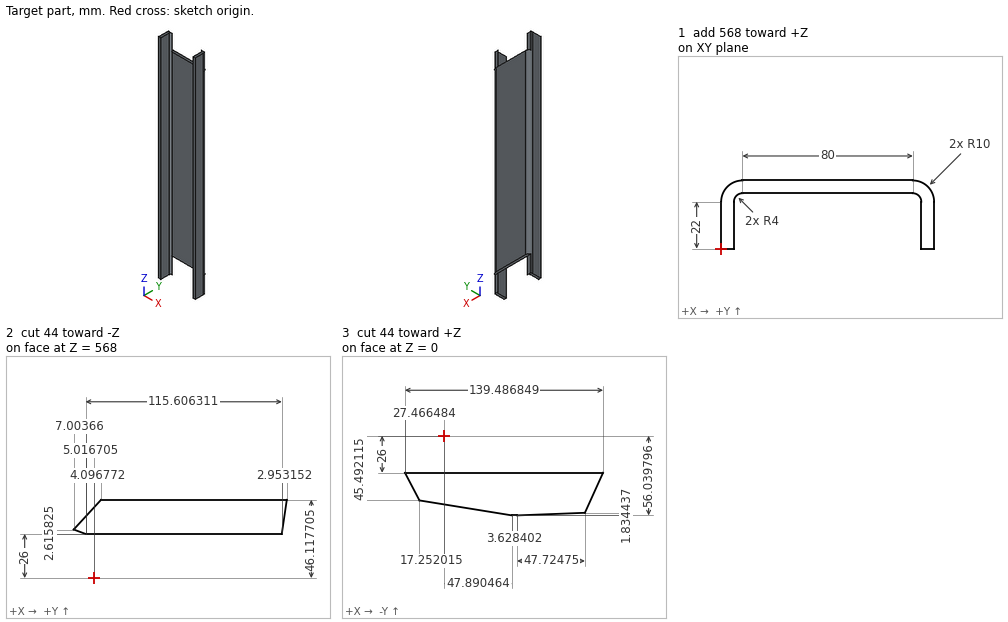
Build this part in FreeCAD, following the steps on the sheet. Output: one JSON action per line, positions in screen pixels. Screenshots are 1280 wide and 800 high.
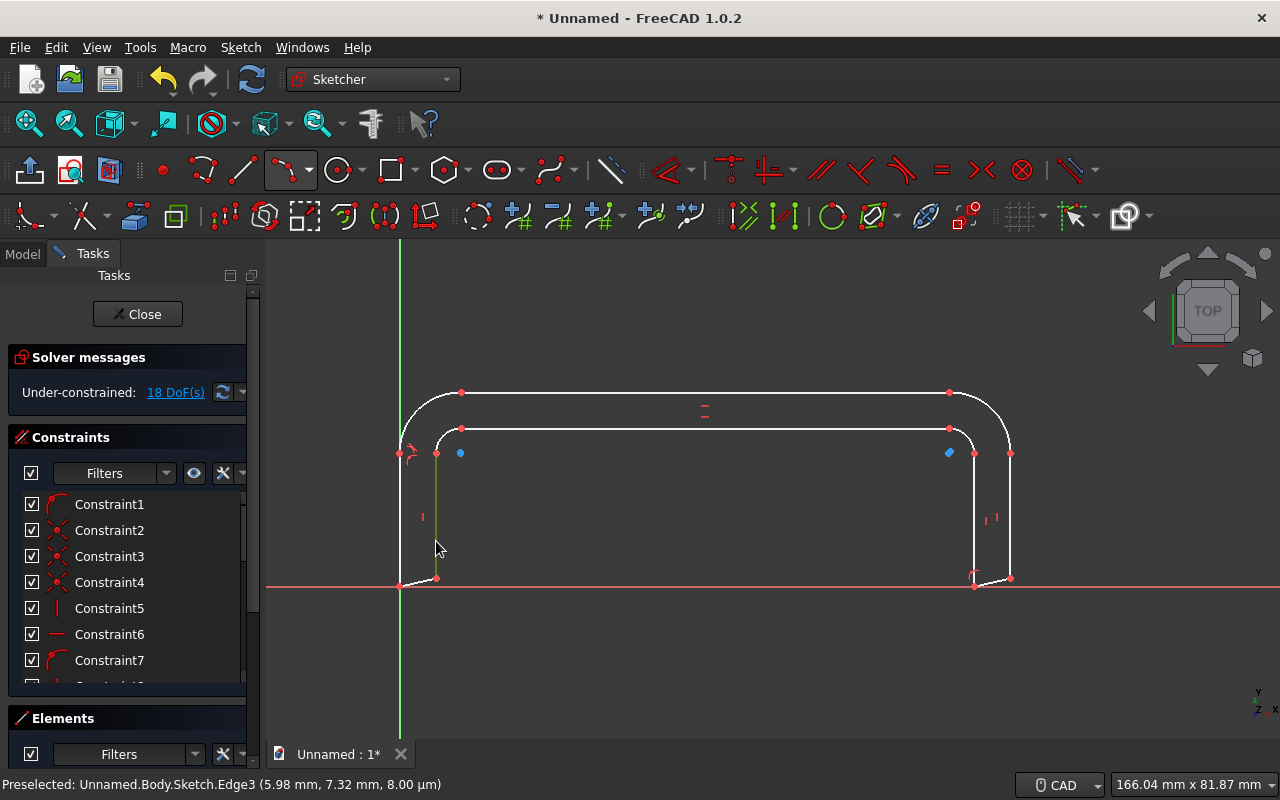
{"action": "left_click", "coordinate": [450, 431]}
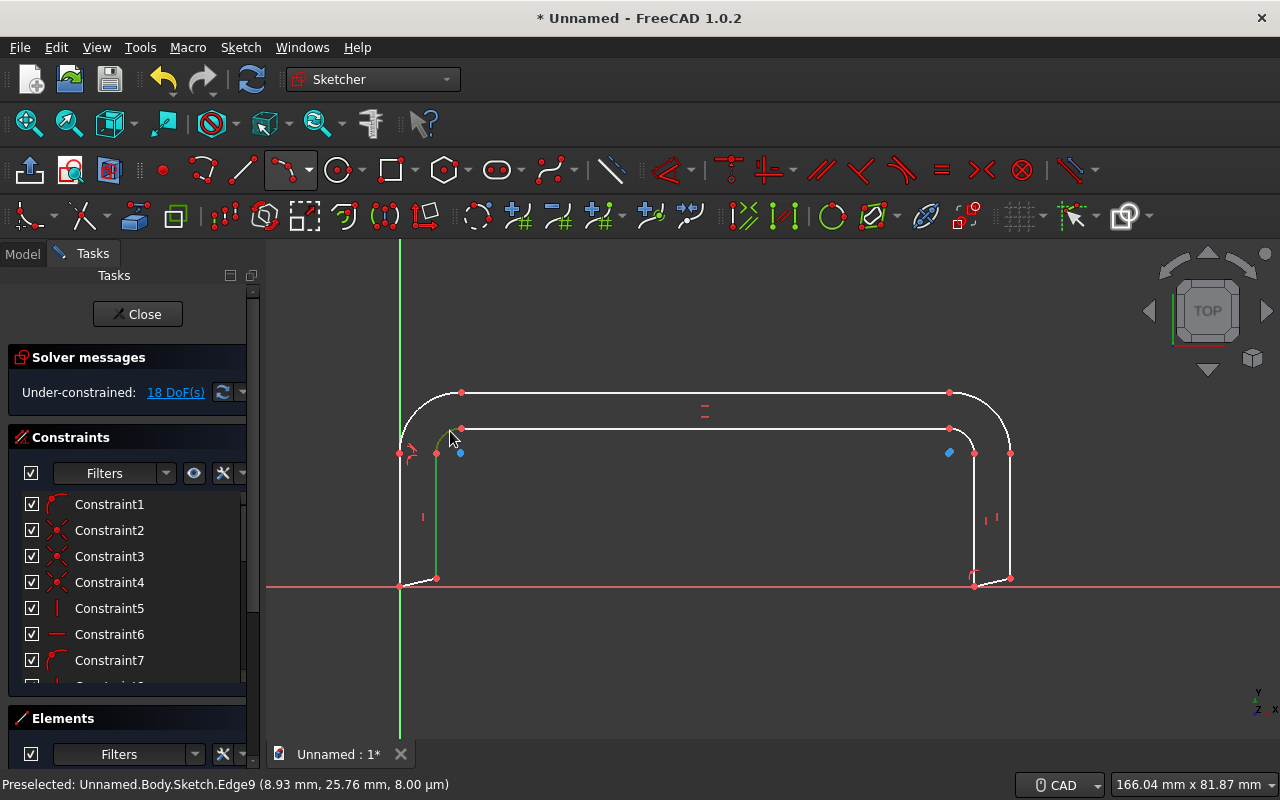
{"action": "left_click", "coordinate": [902, 170]}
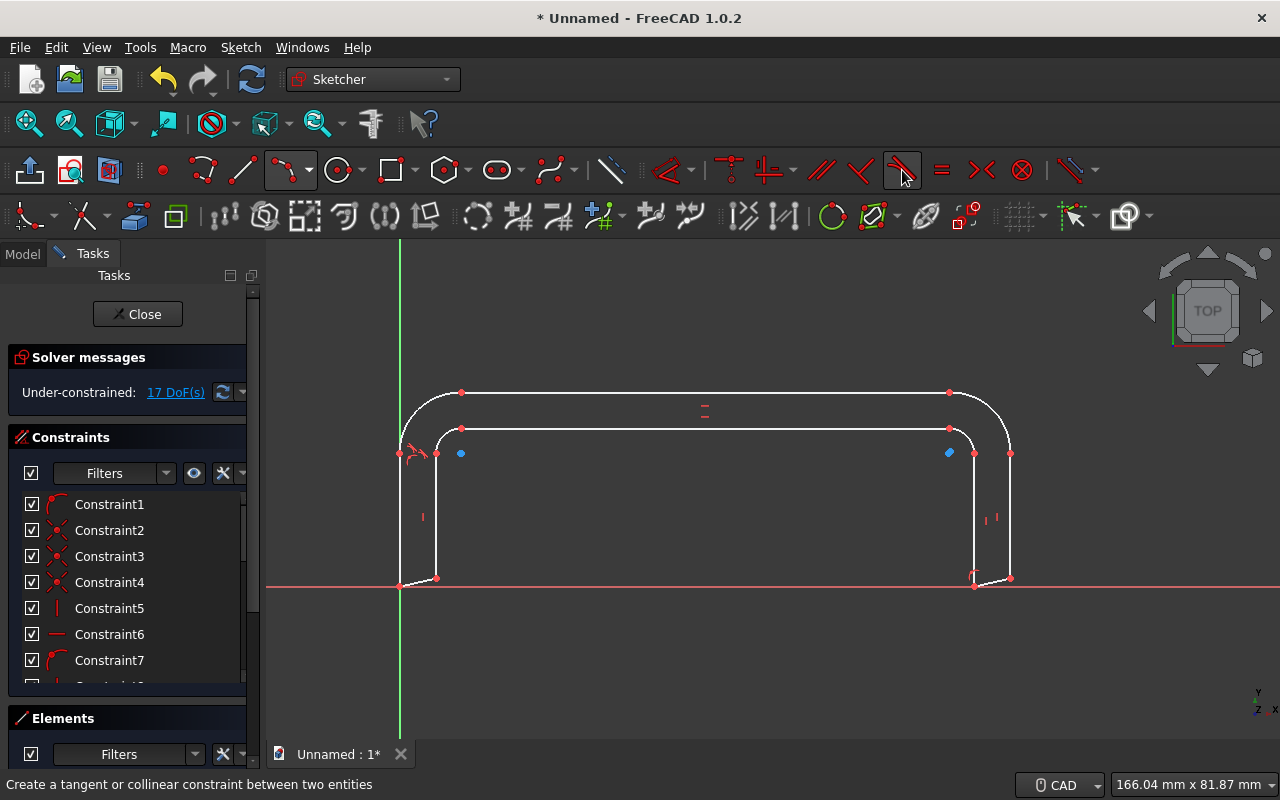
{"action": "left_click", "coordinate": [608, 429]}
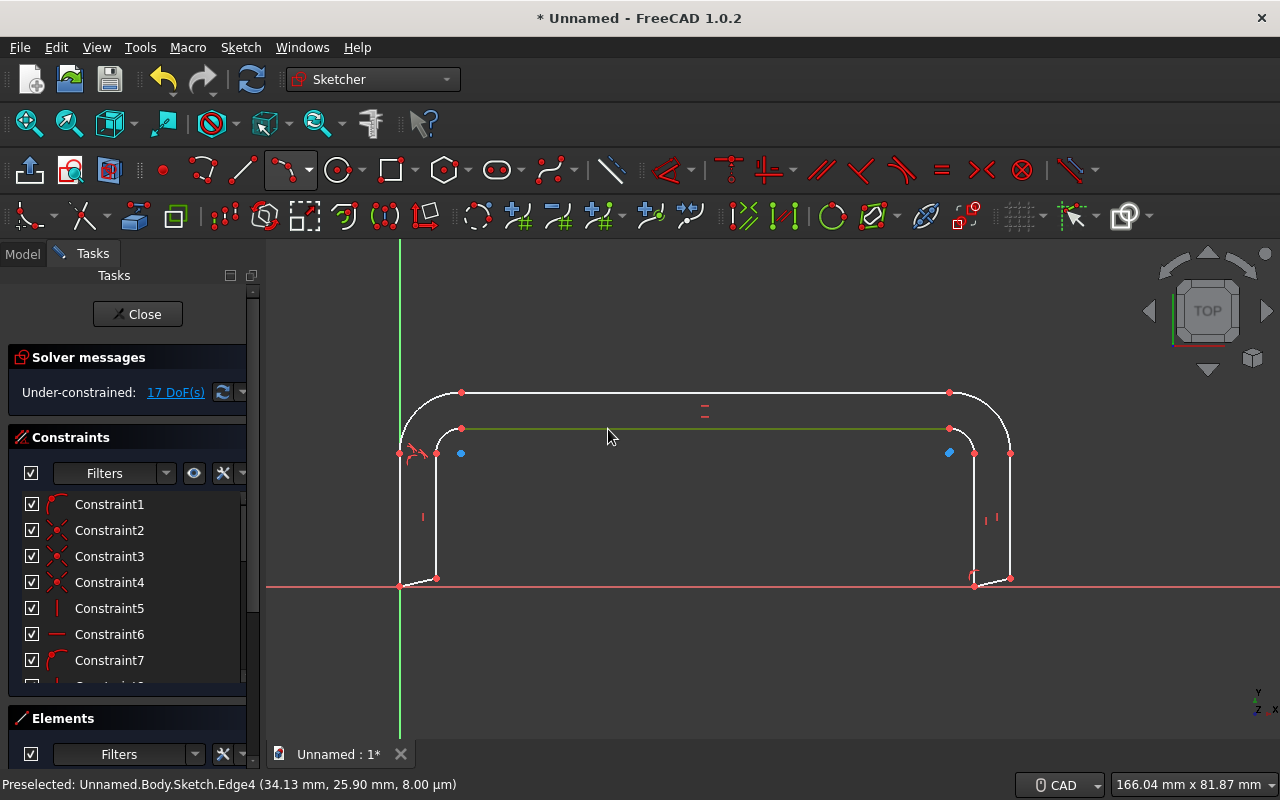
{"action": "left_click", "coordinate": [450, 431]}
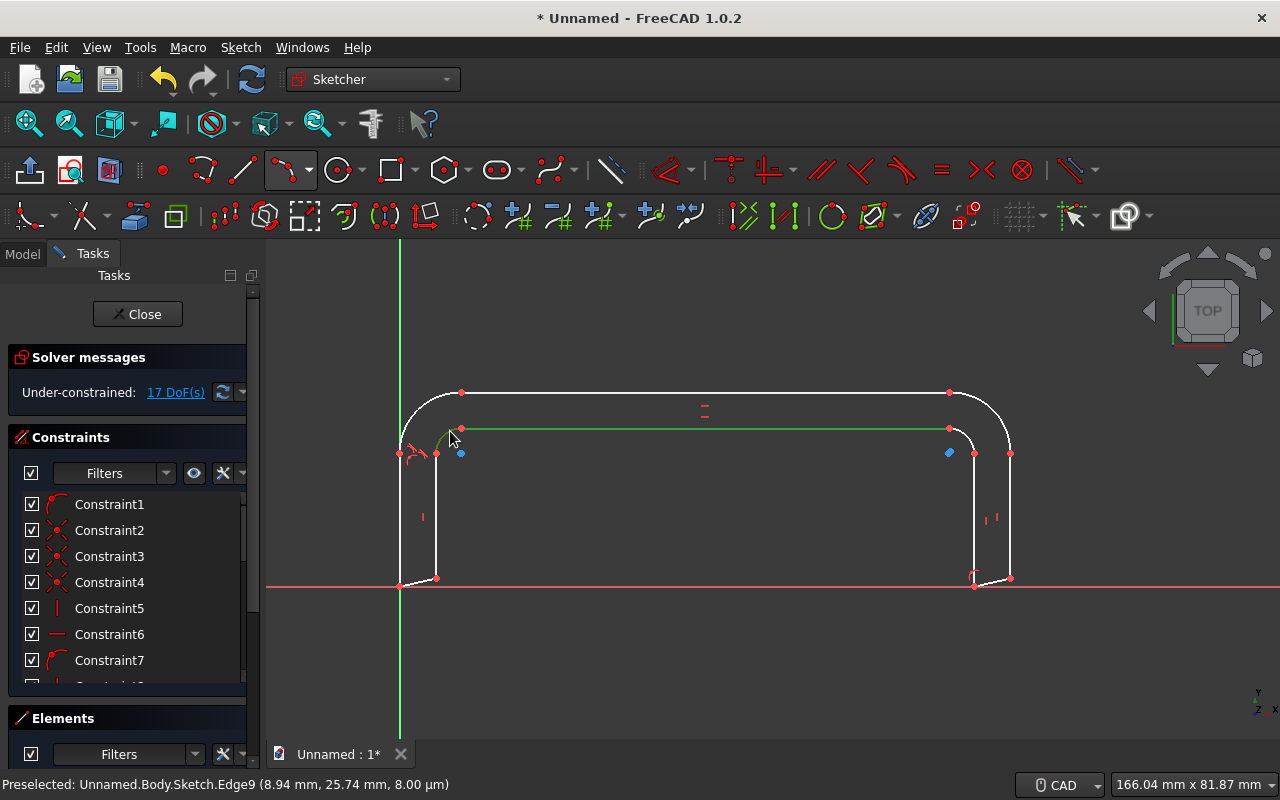
{"action": "left_click", "coordinate": [902, 170]}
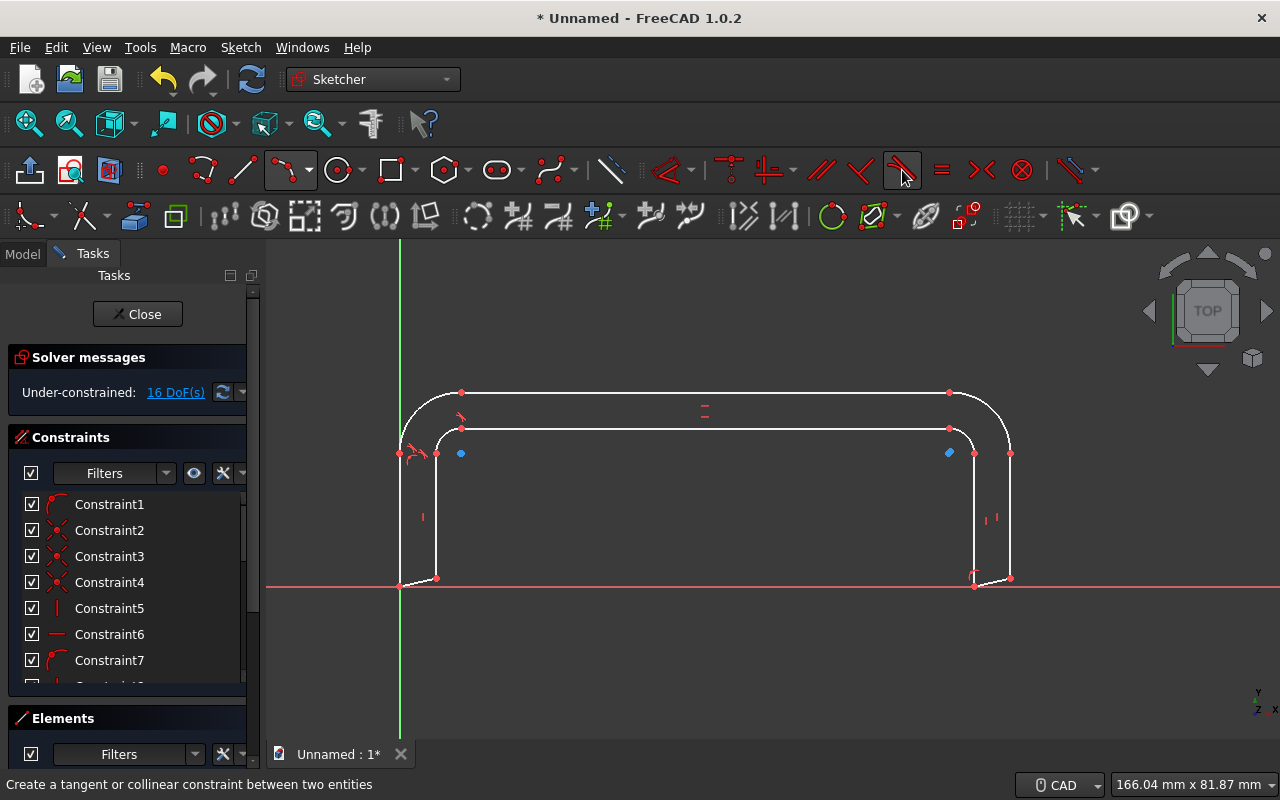
{"action": "left_click", "coordinate": [608, 429]}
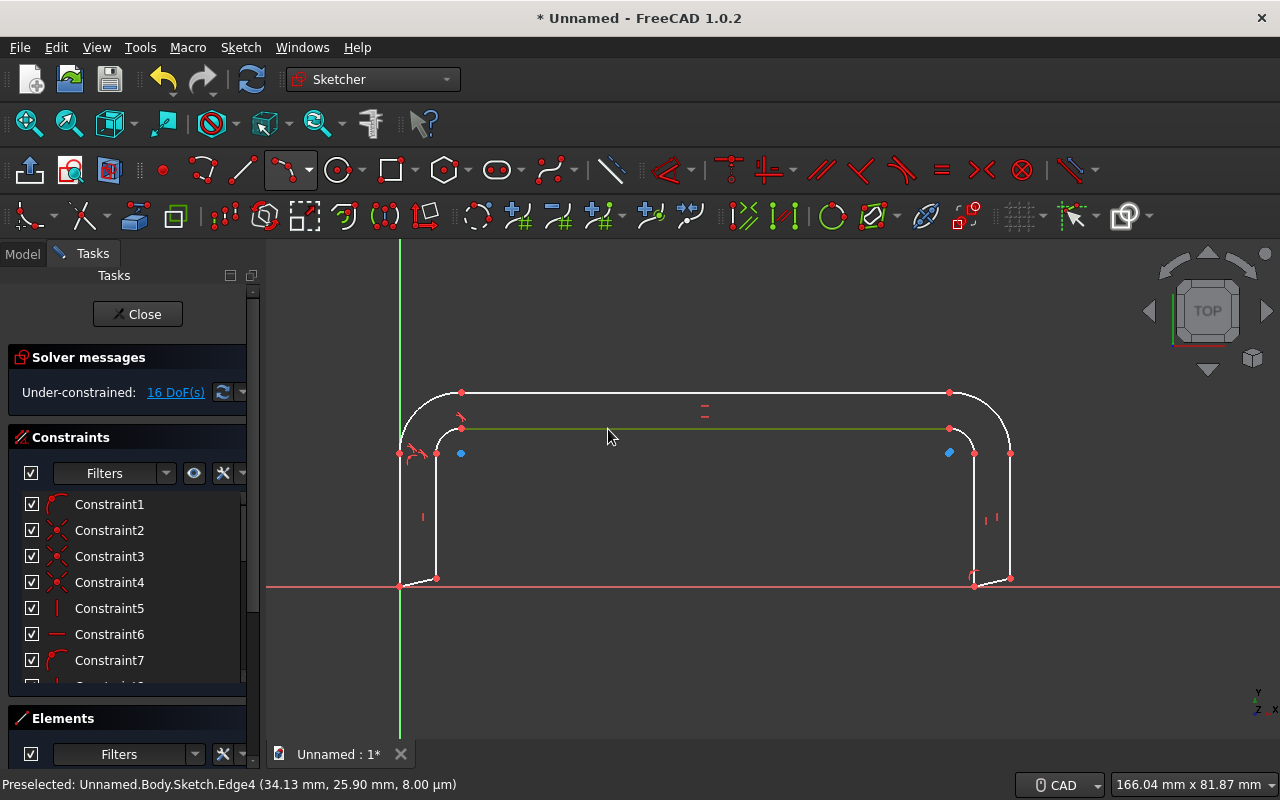
{"action": "left_click", "coordinate": [971, 442]}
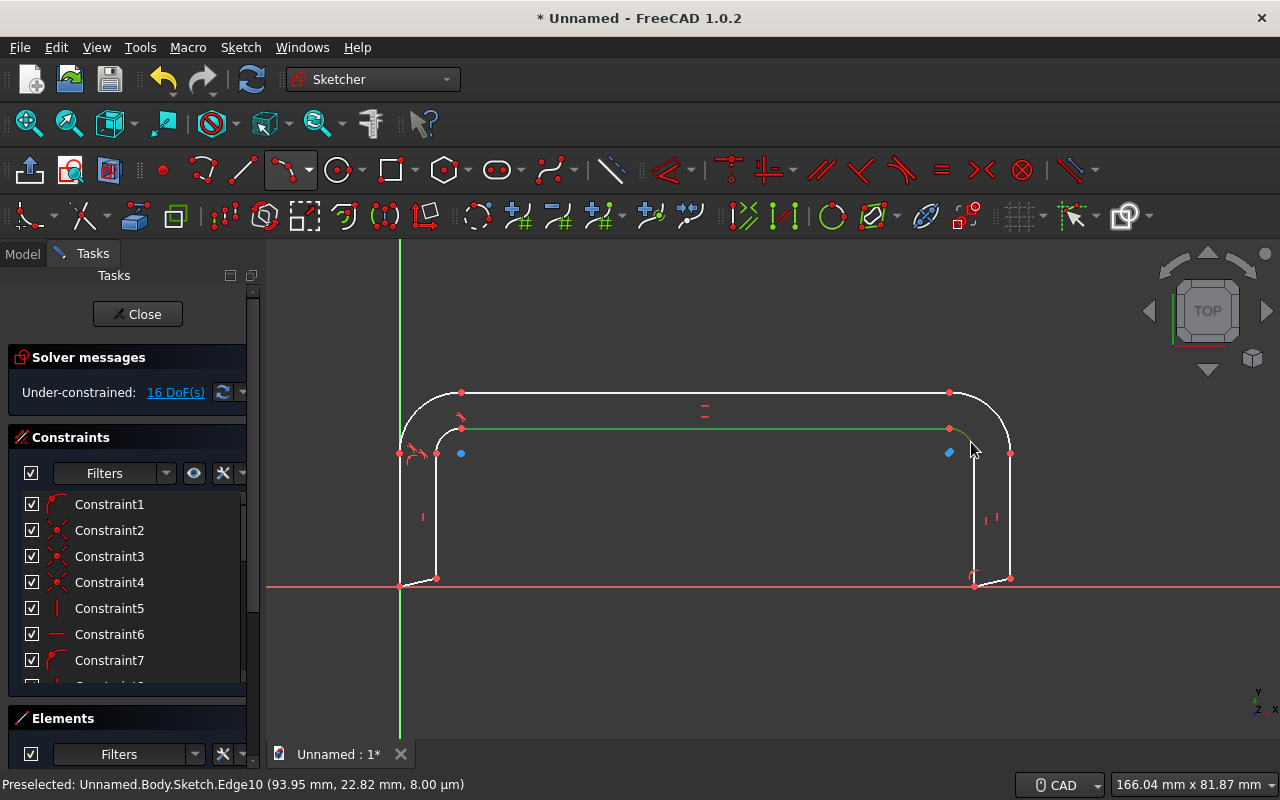
{"action": "left_click", "coordinate": [902, 170]}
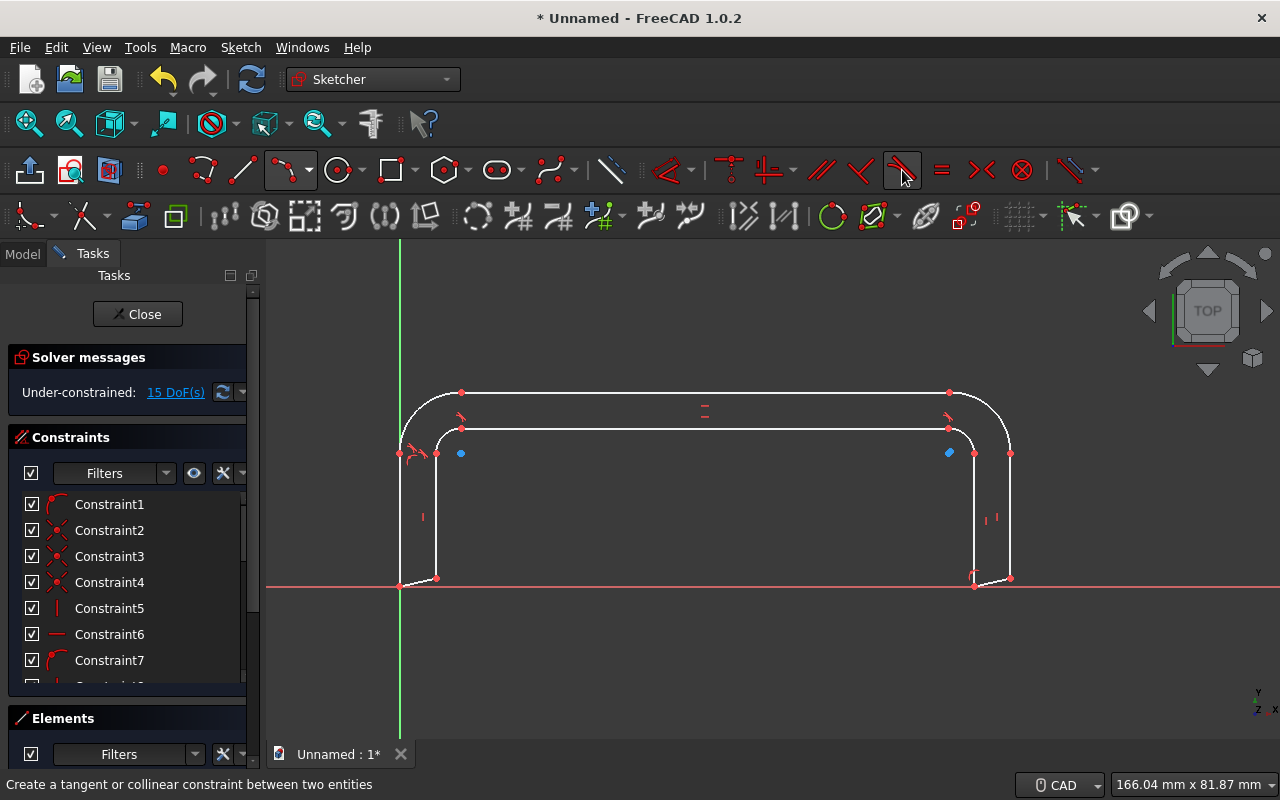
{"action": "left_click", "coordinate": [974, 494]}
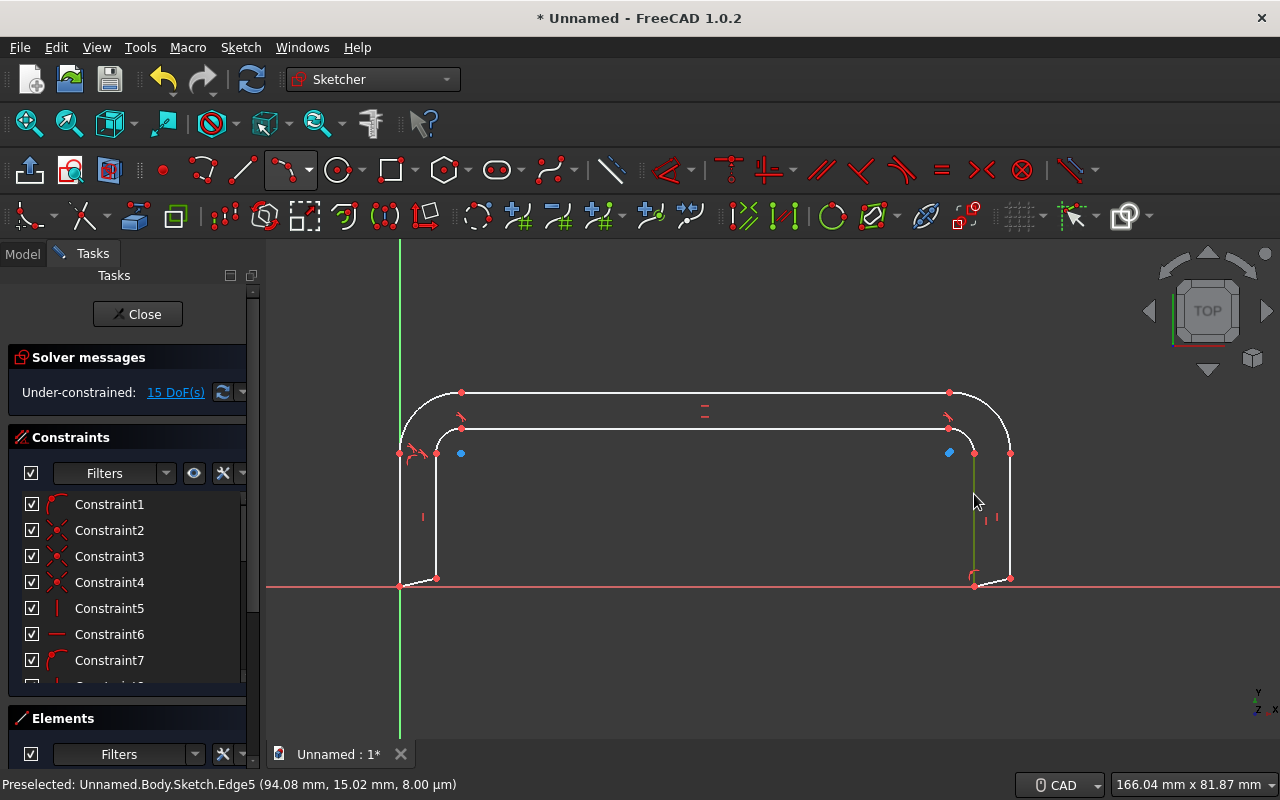
{"action": "left_click", "coordinate": [971, 442]}